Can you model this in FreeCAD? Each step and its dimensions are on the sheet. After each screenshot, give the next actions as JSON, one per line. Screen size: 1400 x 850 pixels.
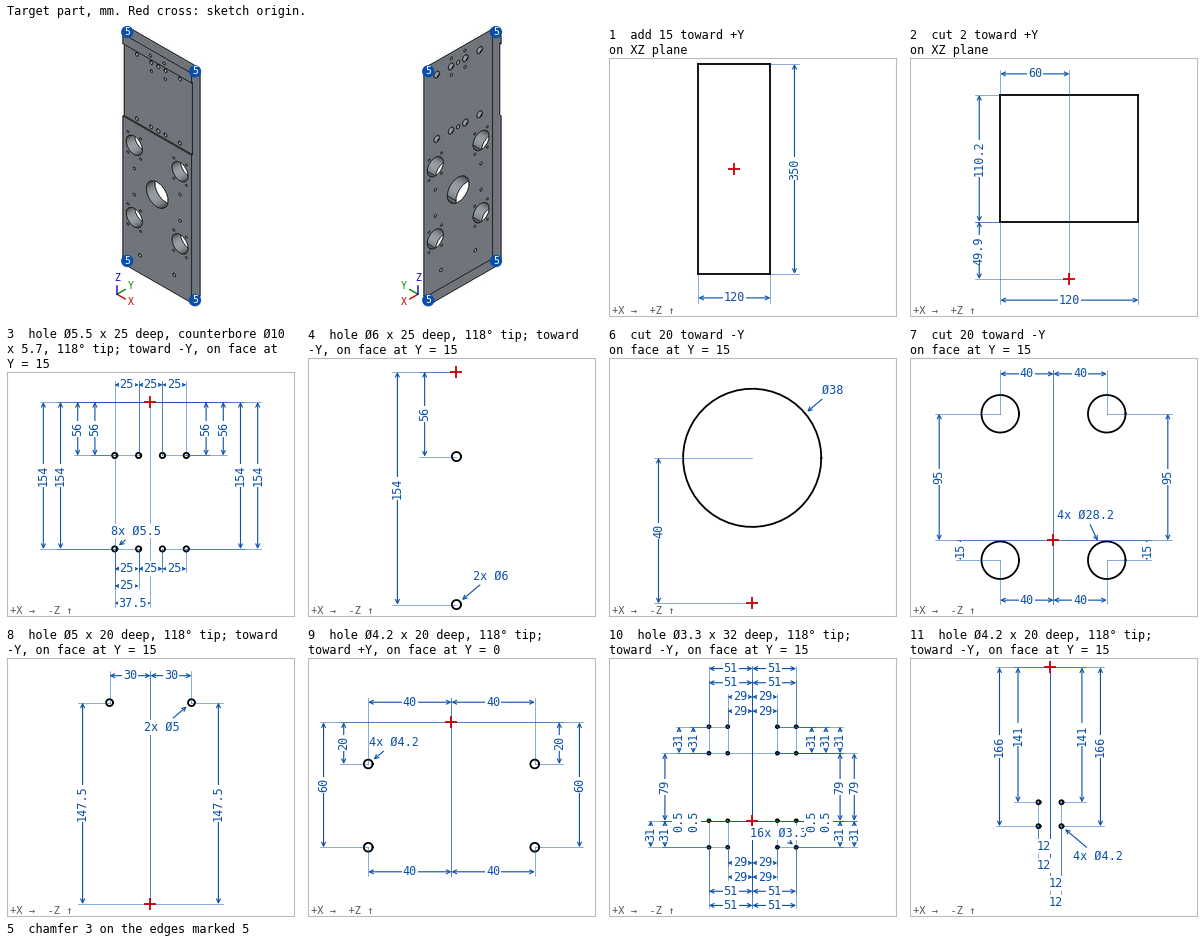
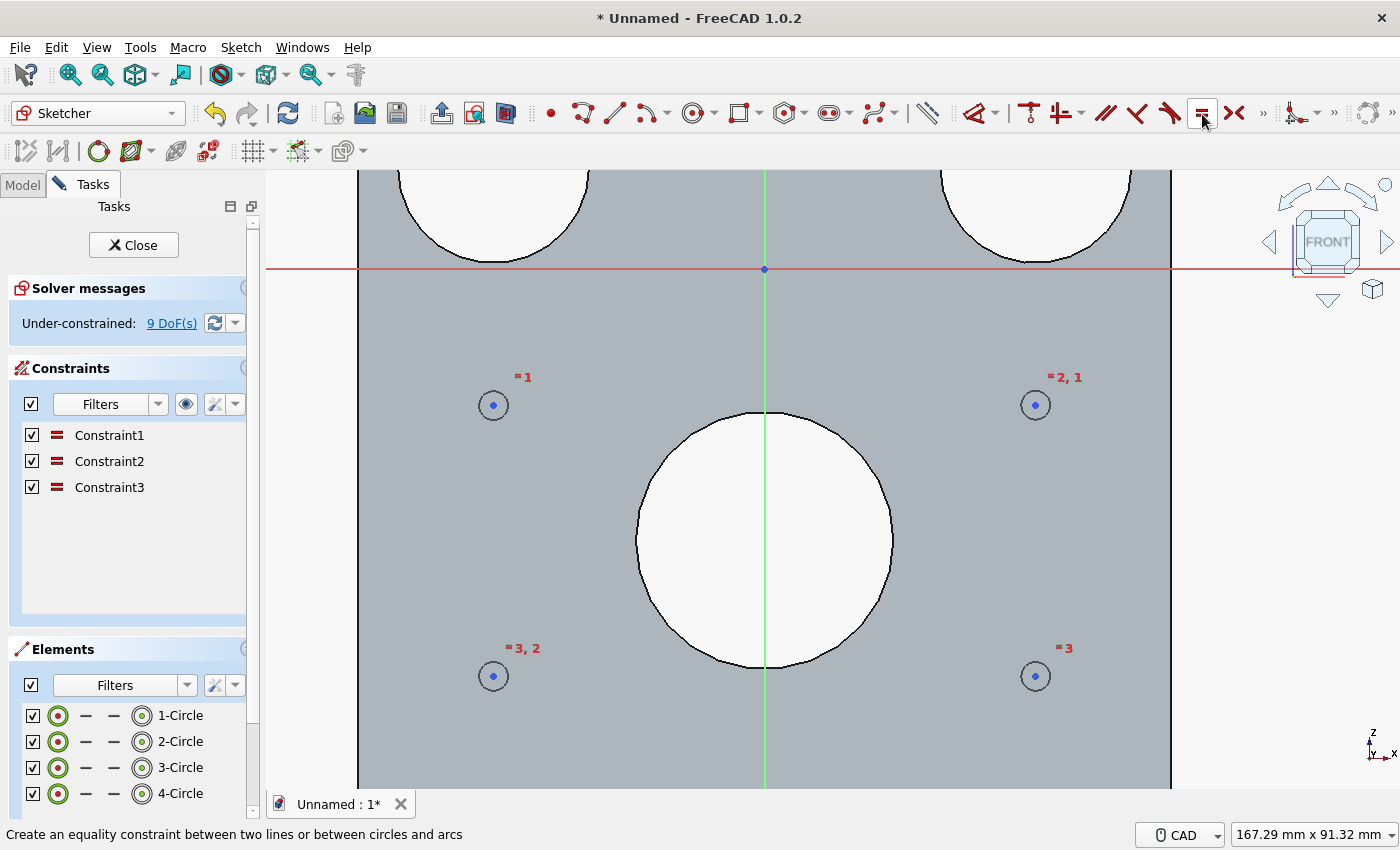
{"action": "left_click", "coordinate": [974, 114]}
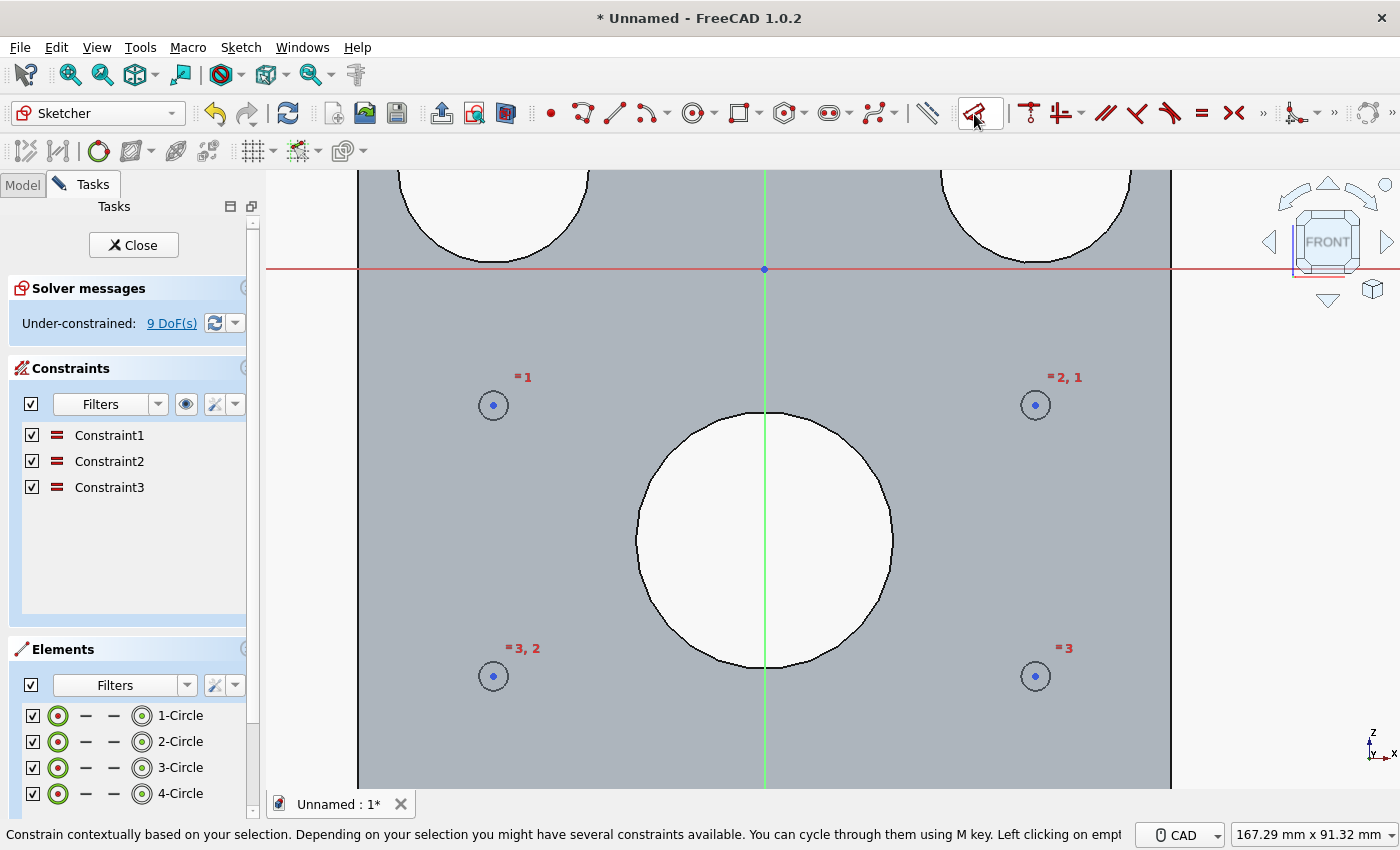
{"action": "scroll", "coordinate": [504, 395], "scroll_direction": "up", "scroll_amount": 2}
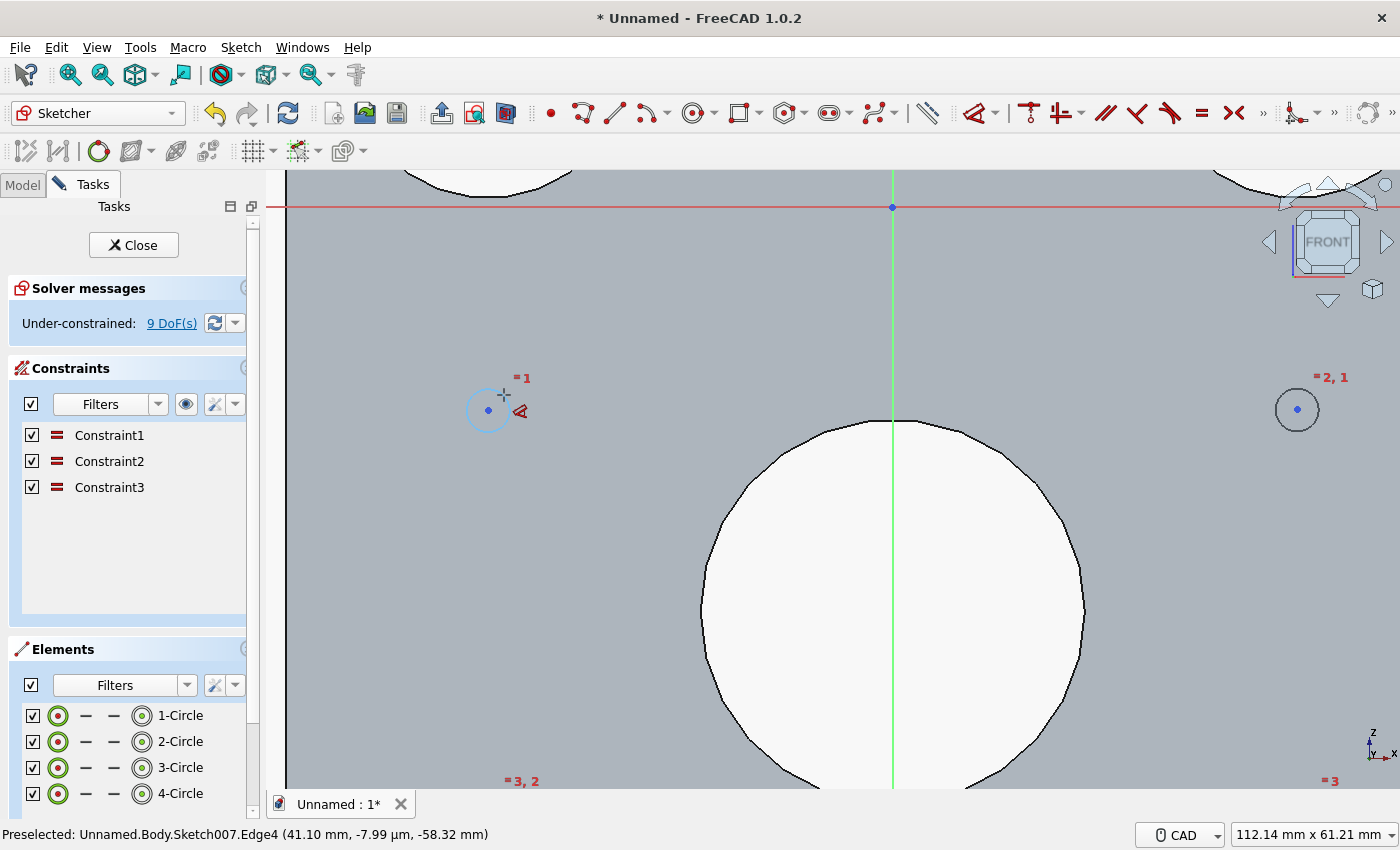
{"action": "left_click", "coordinate": [503, 395]}
{"action": "left_click", "coordinate": [525, 372]}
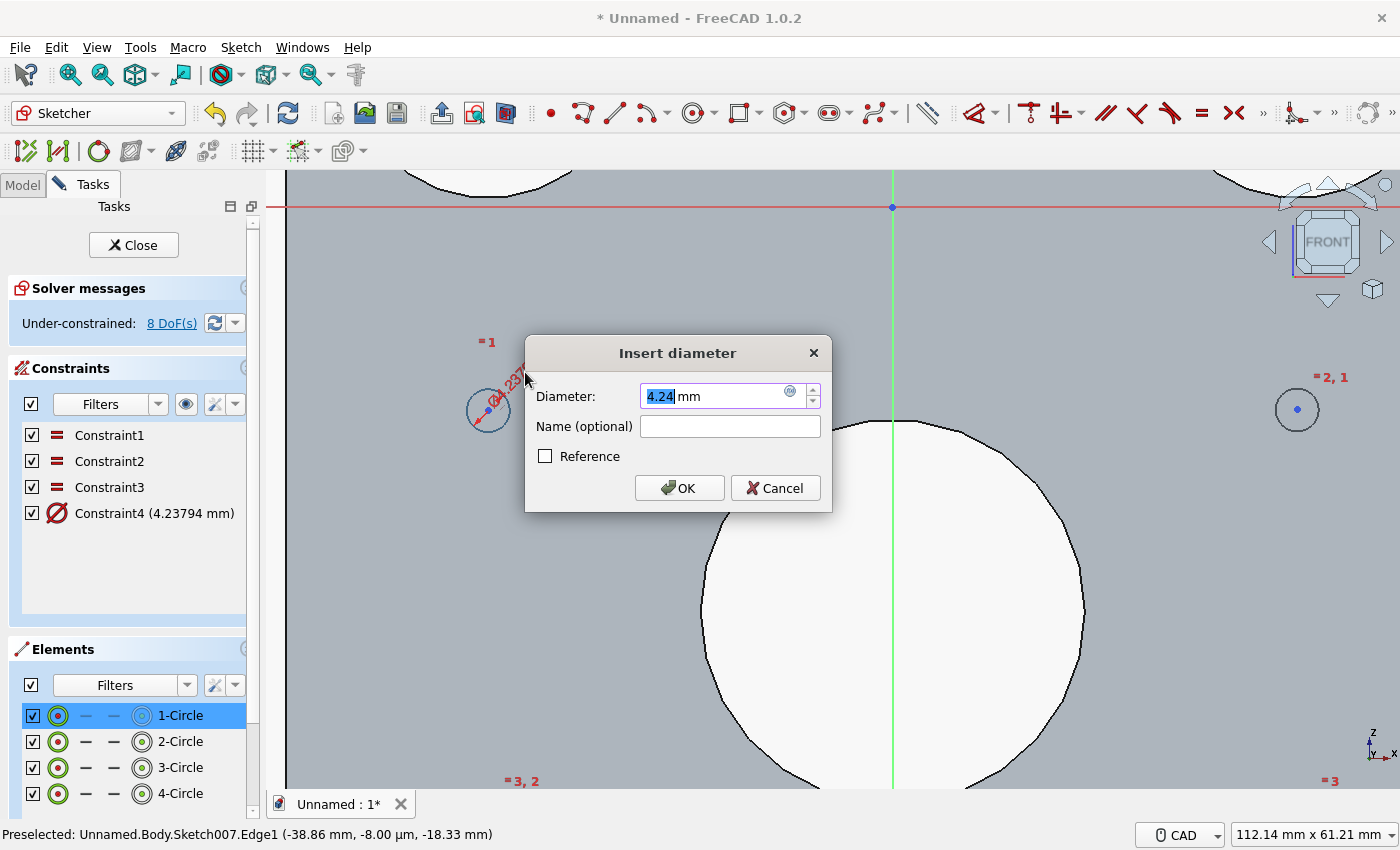
{"action": "type", "text": "4.2"}
{"action": "key", "text": "Return"}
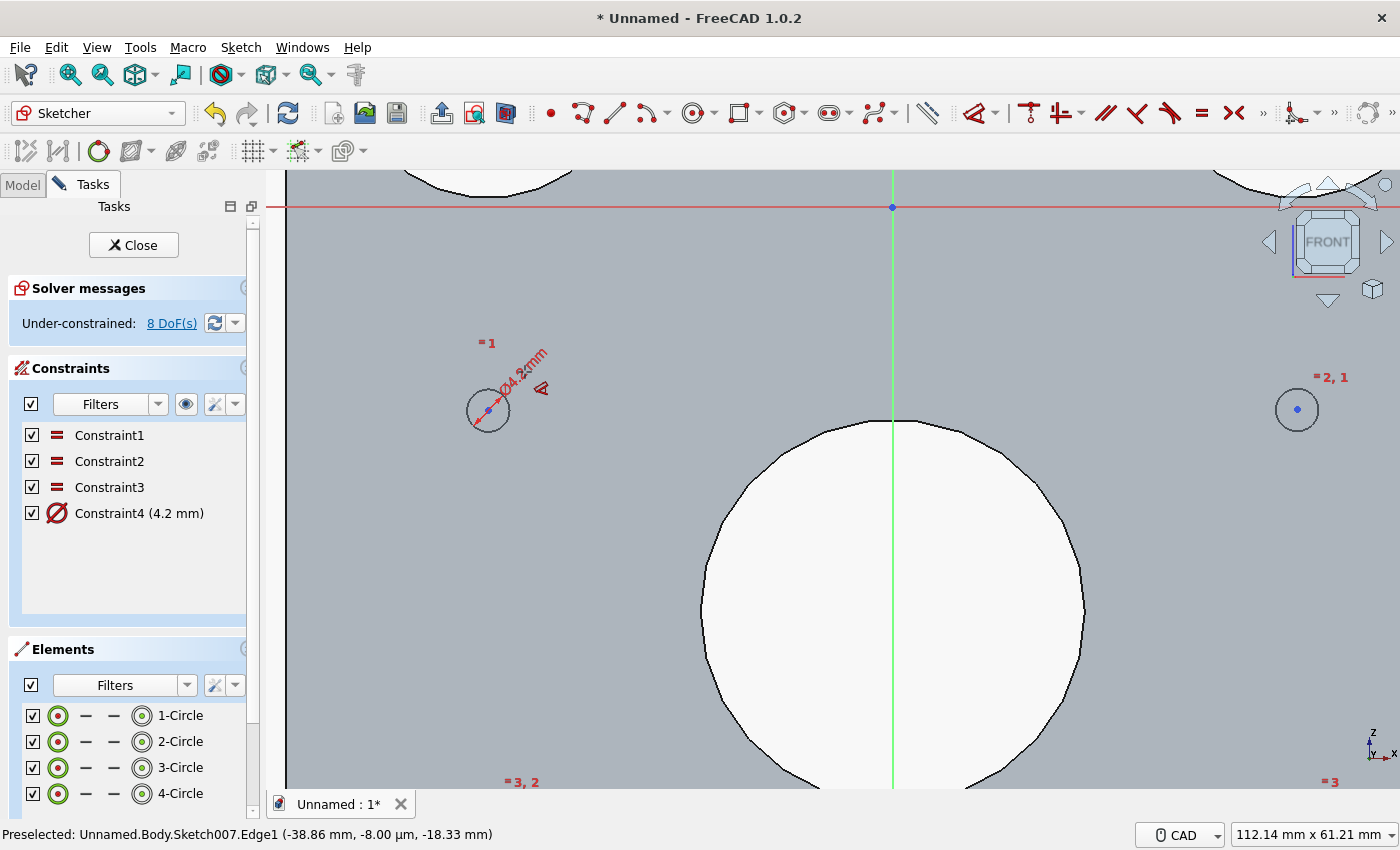
{"action": "left_click", "coordinate": [488, 411]}
{"action": "left_click", "coordinate": [691, 445]}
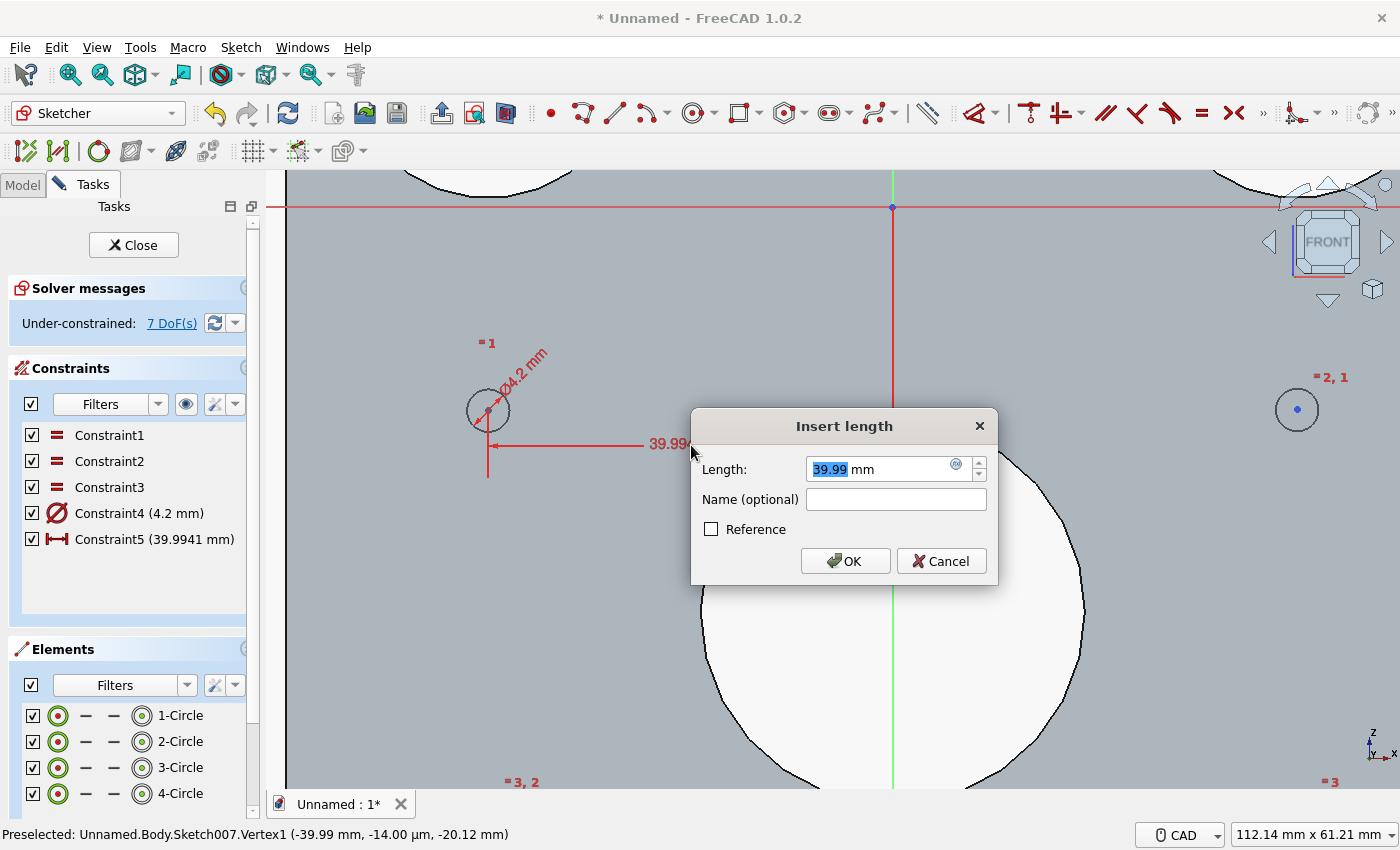
{"action": "type", "text": "40"}
{"action": "key", "text": "Return"}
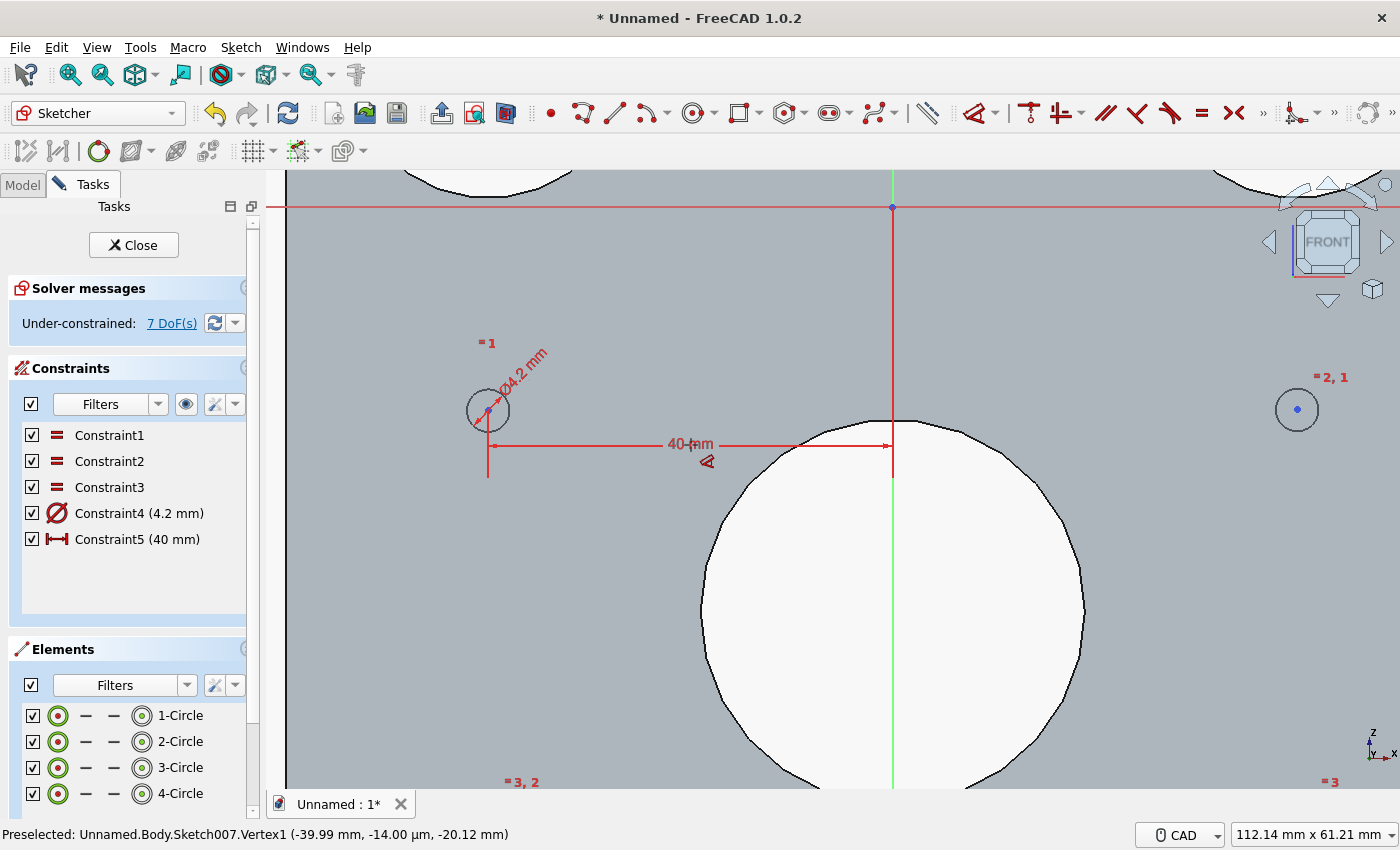
{"action": "left_click", "coordinate": [488, 411]}
{"action": "left_click", "coordinate": [454, 309]}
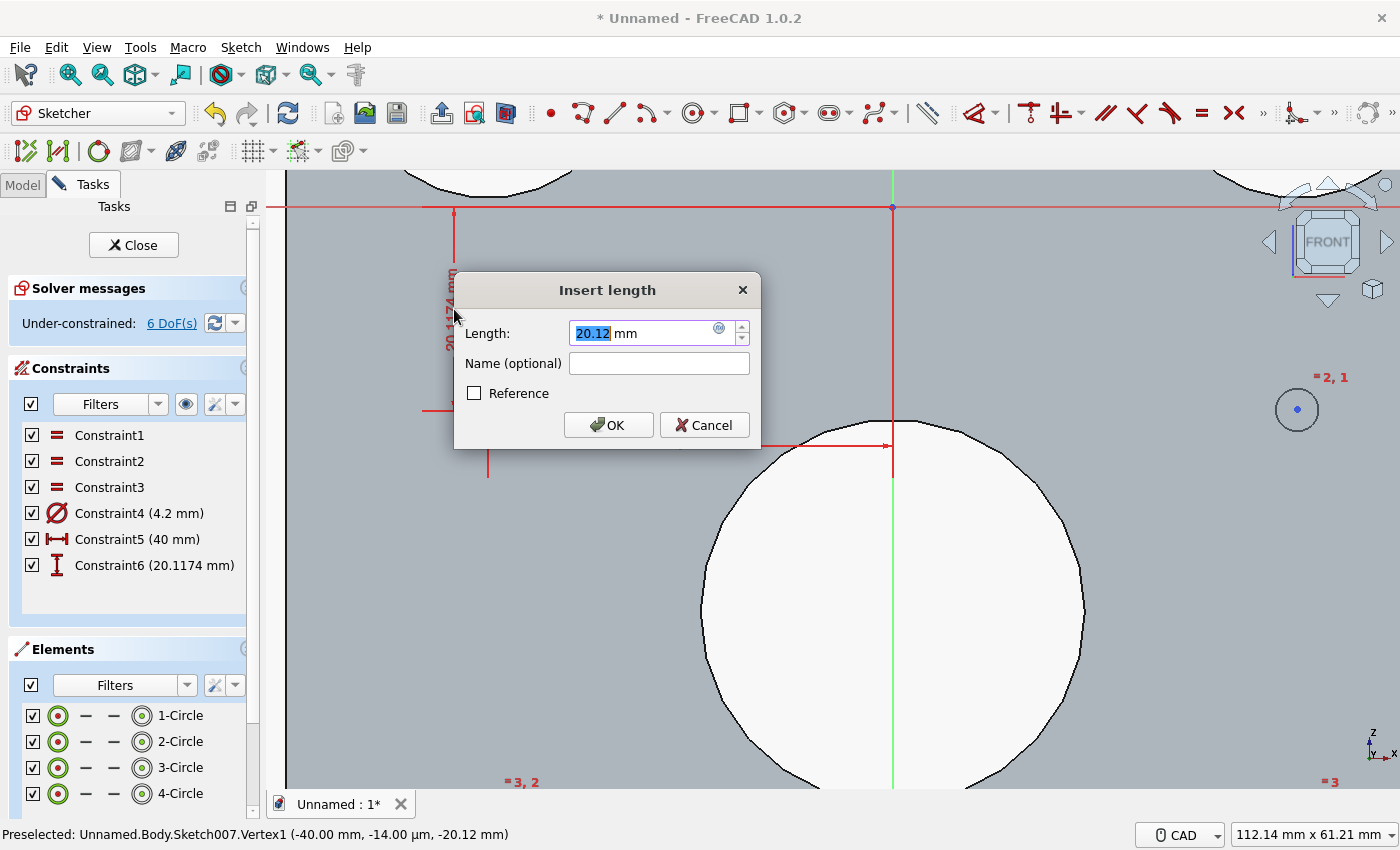
{"action": "type", "text": "20"}
{"action": "key", "text": "Return"}